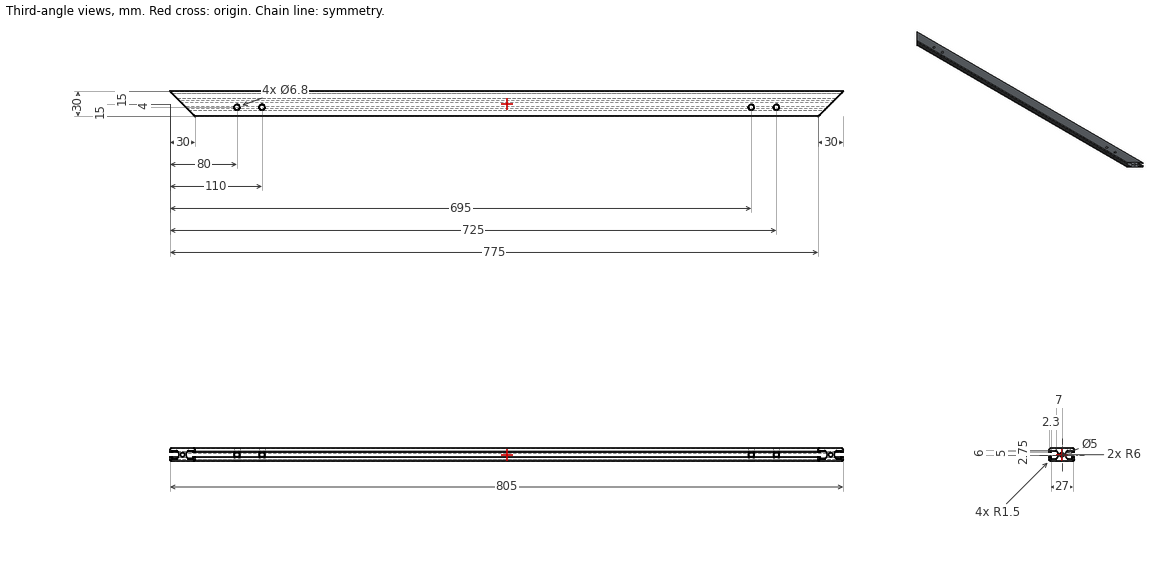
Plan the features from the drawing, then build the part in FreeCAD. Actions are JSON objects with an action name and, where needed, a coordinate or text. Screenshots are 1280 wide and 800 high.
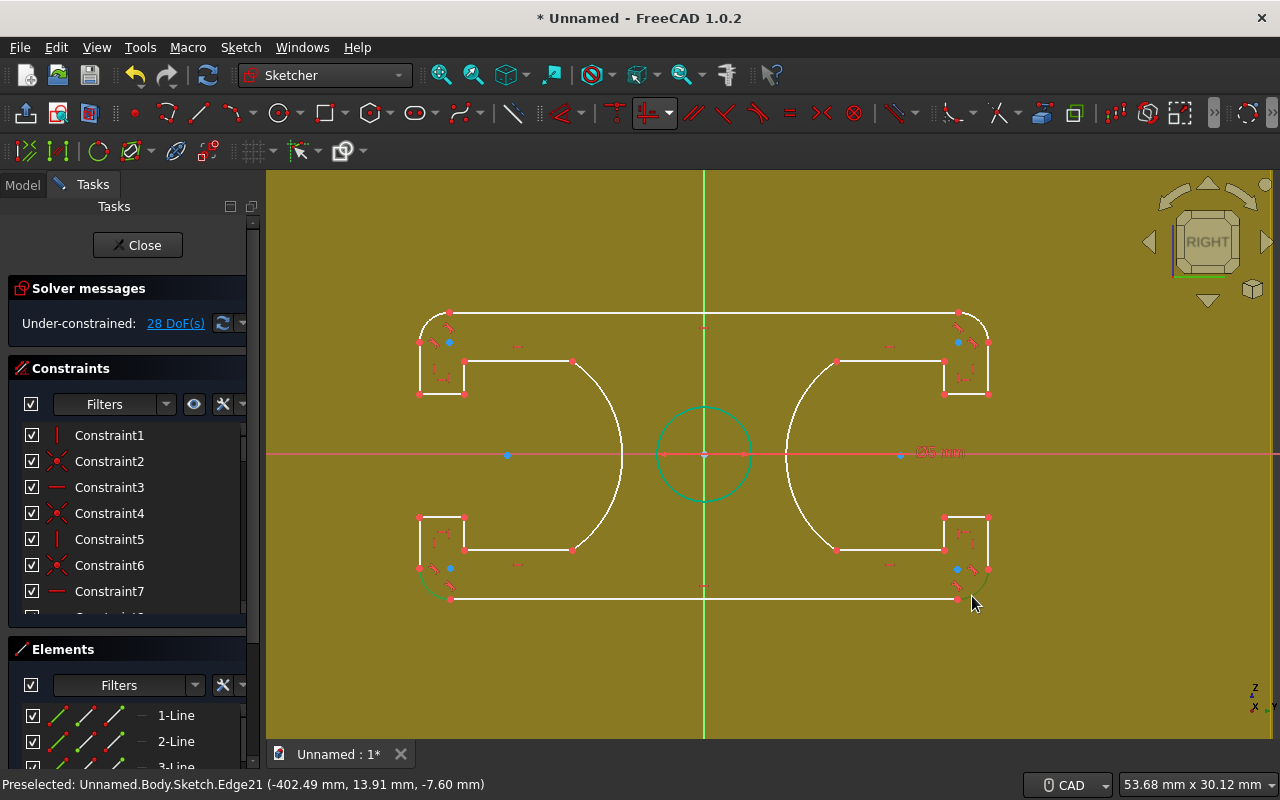
{"action": "left_click", "coordinate": [985, 329]}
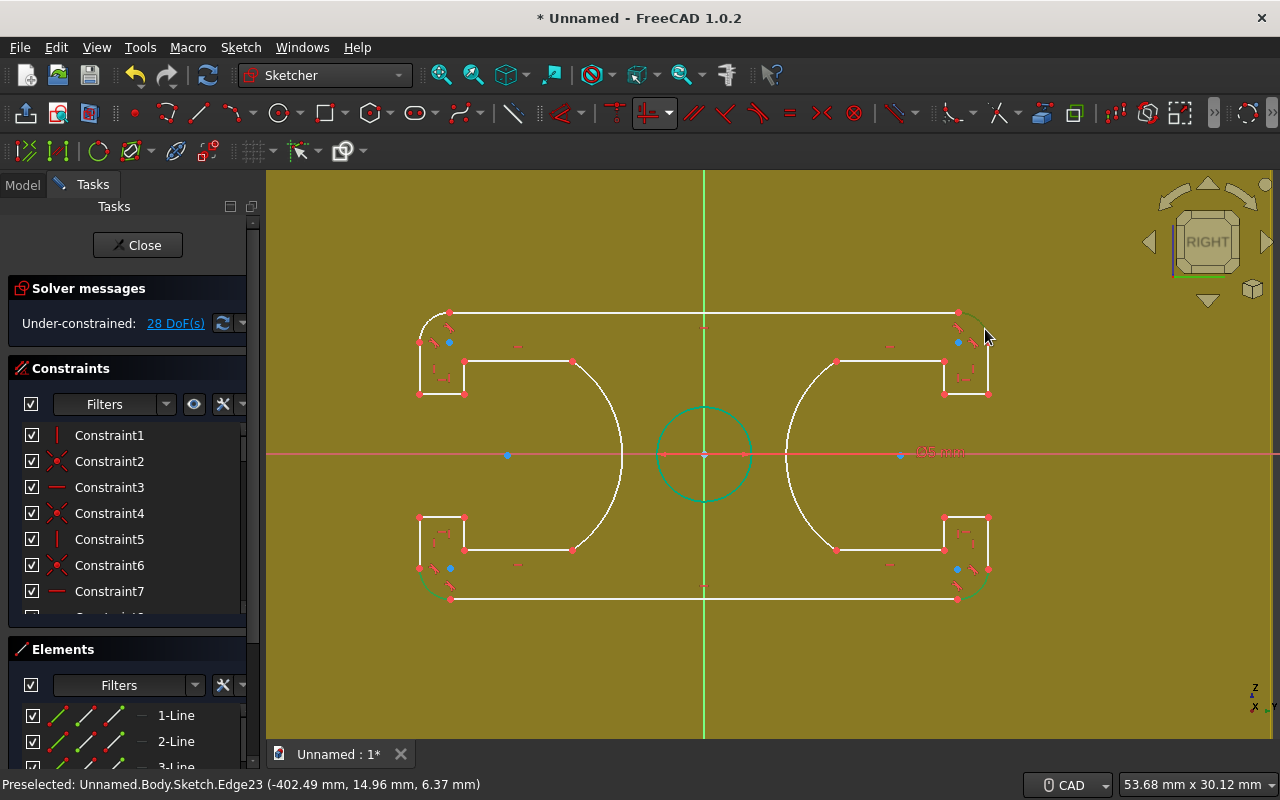
{"action": "left_click", "coordinate": [436, 316]}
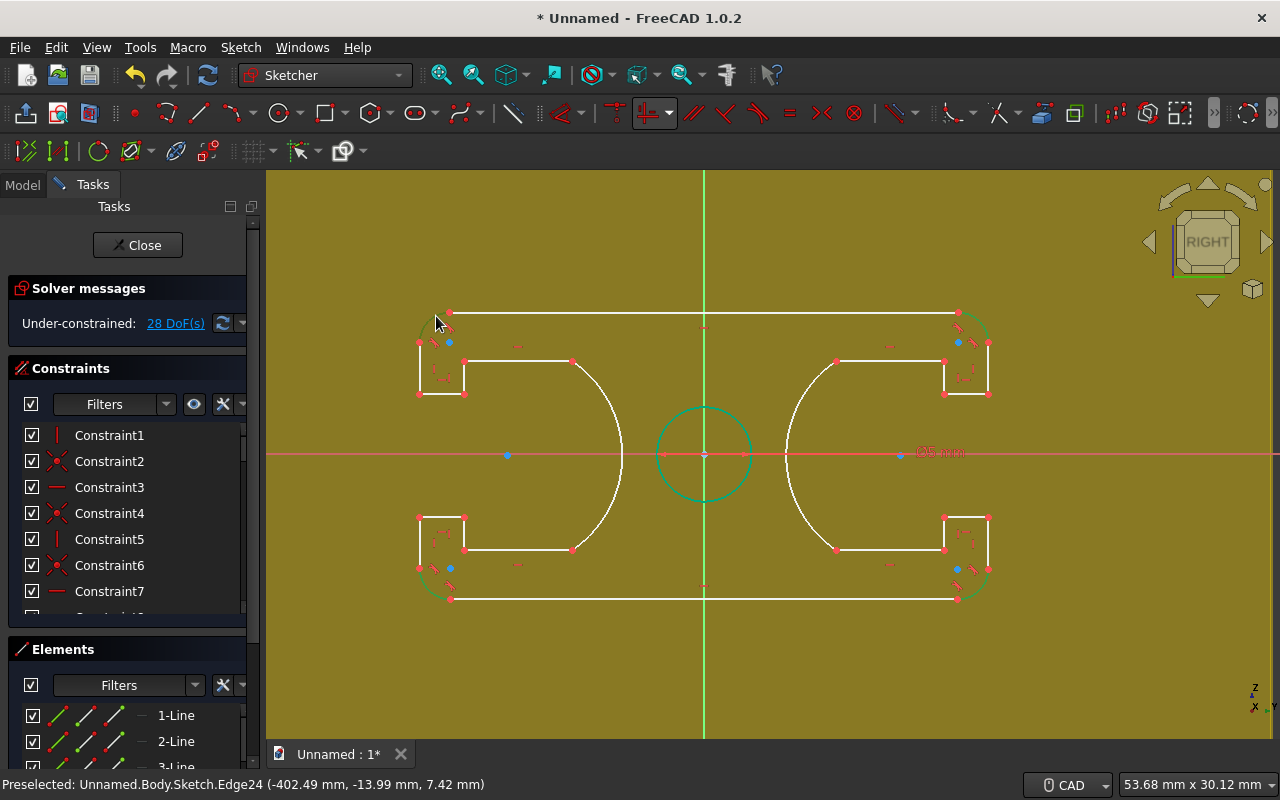
{"action": "left_click", "coordinate": [790, 114]}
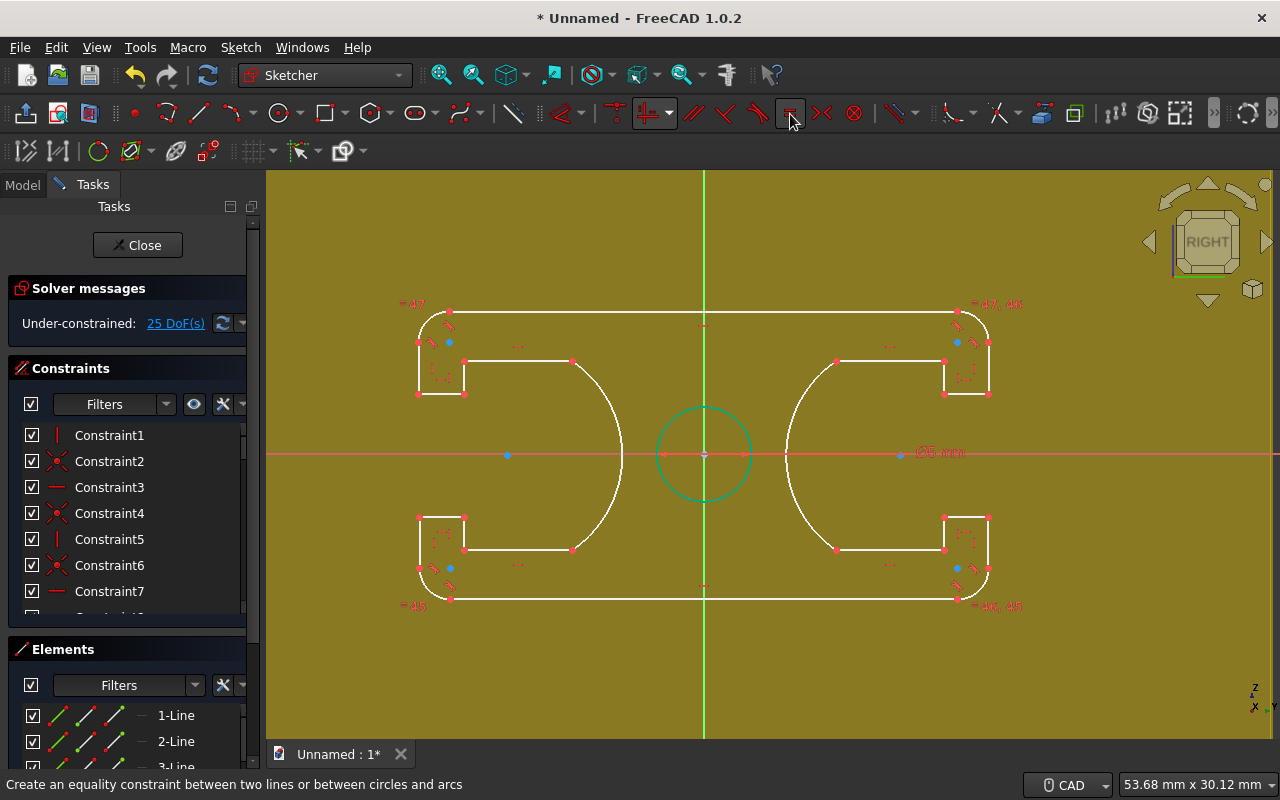
{"action": "left_click", "coordinate": [614, 499]}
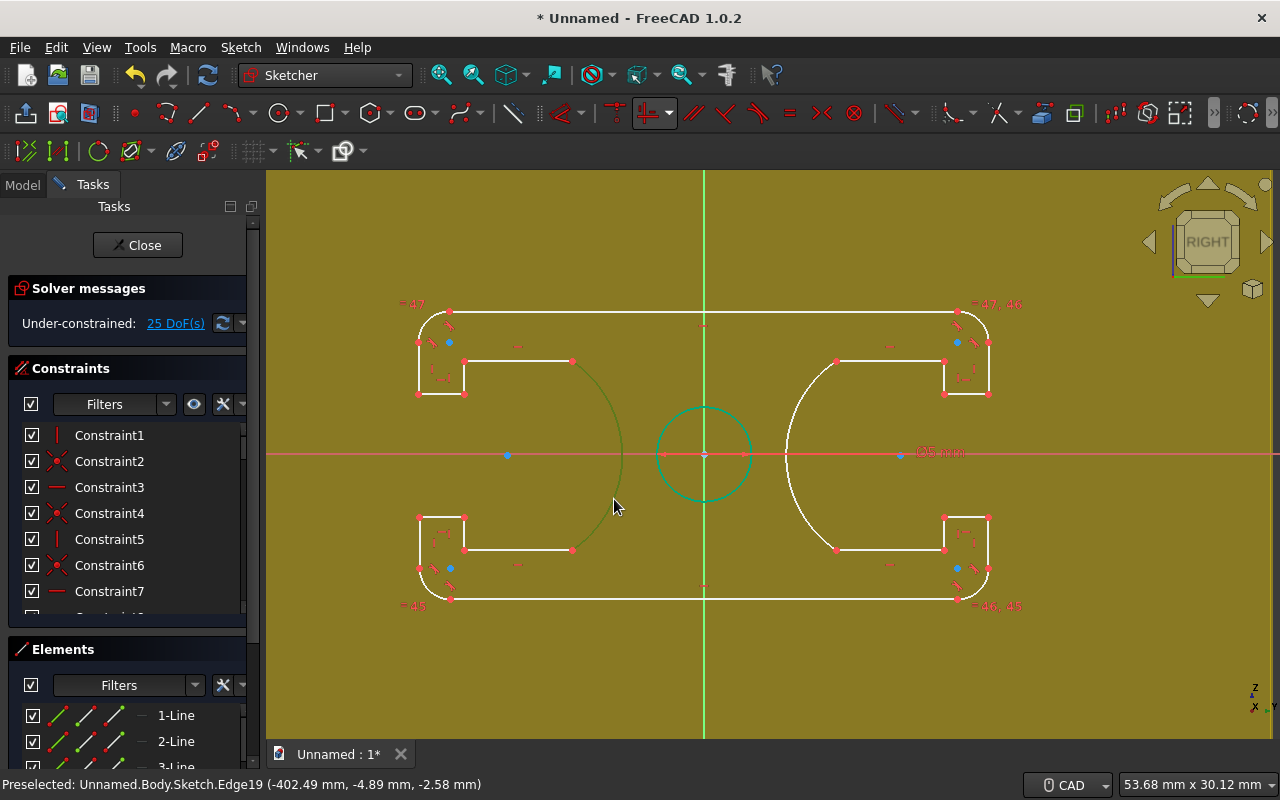
{"action": "left_click", "coordinate": [795, 412]}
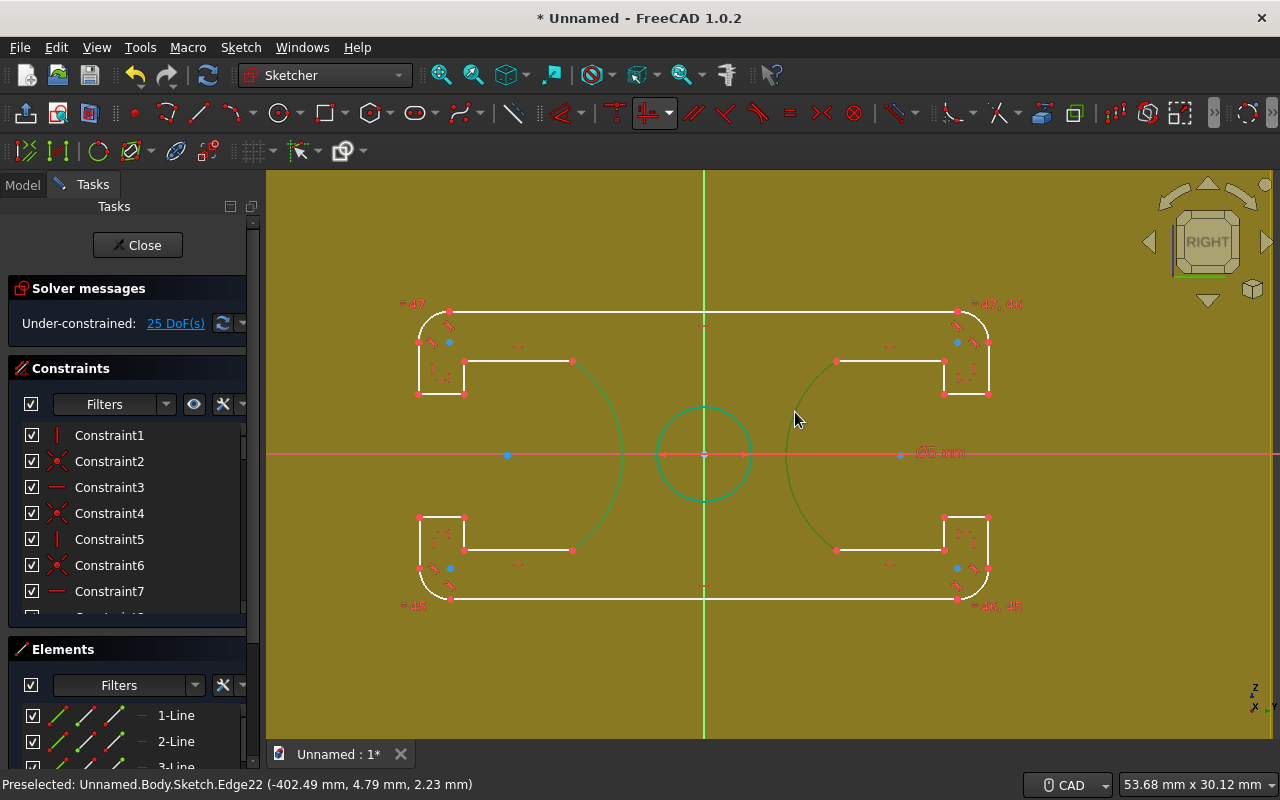
{"action": "left_click", "coordinate": [790, 114]}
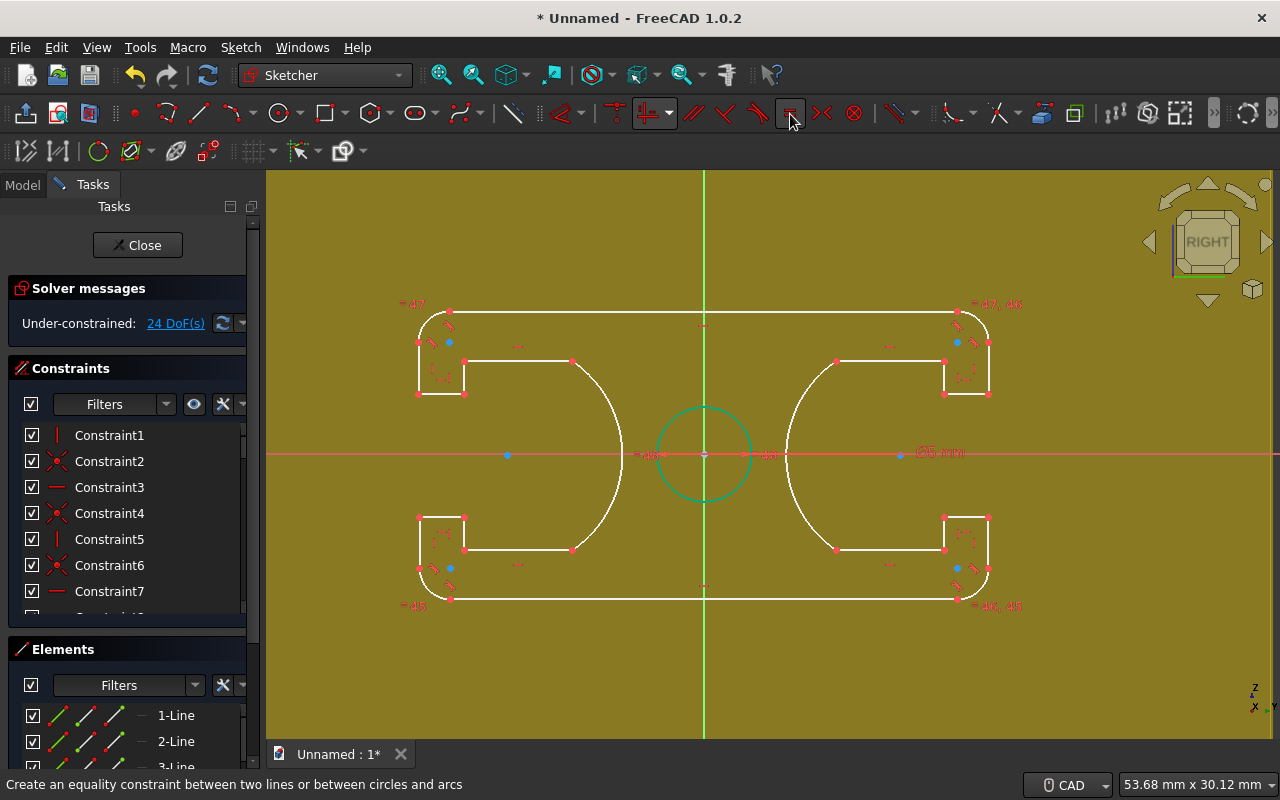
{"action": "left_click", "coordinate": [508, 456]}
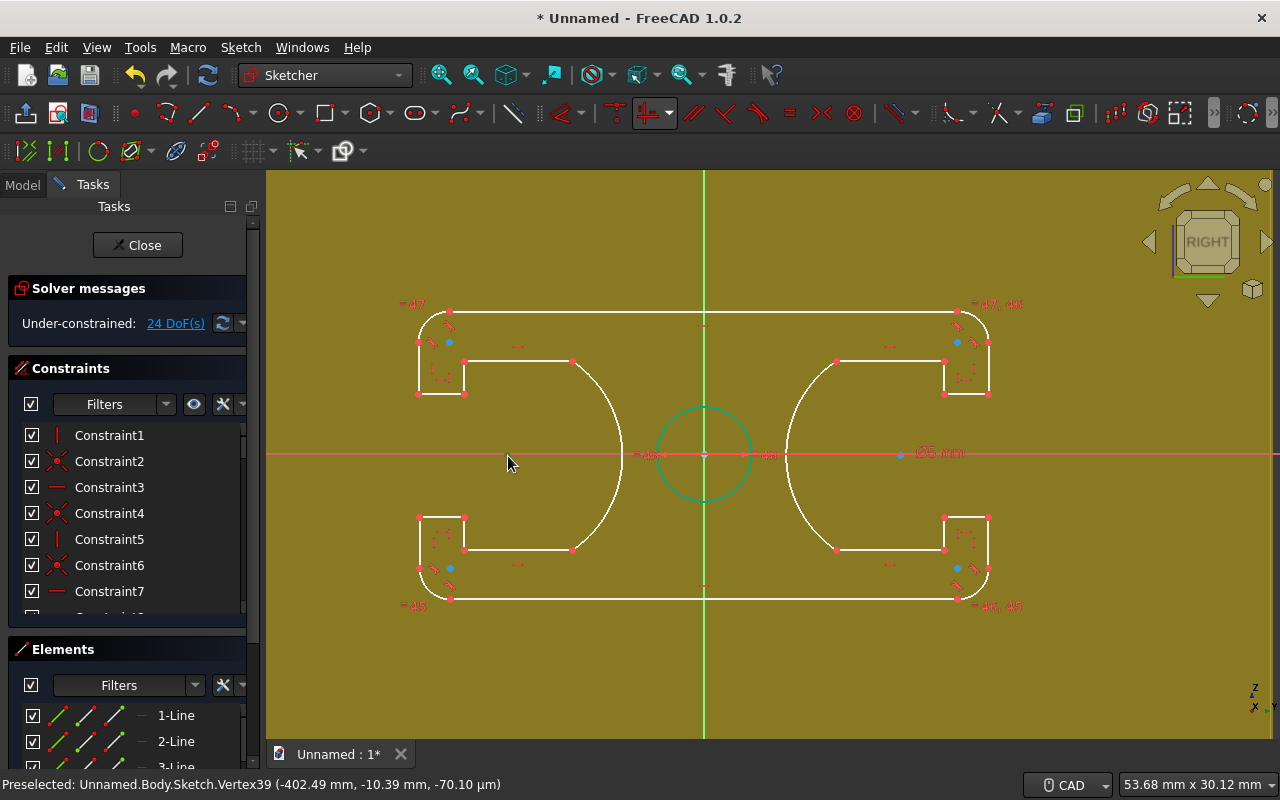
{"action": "left_click", "coordinate": [353, 454]}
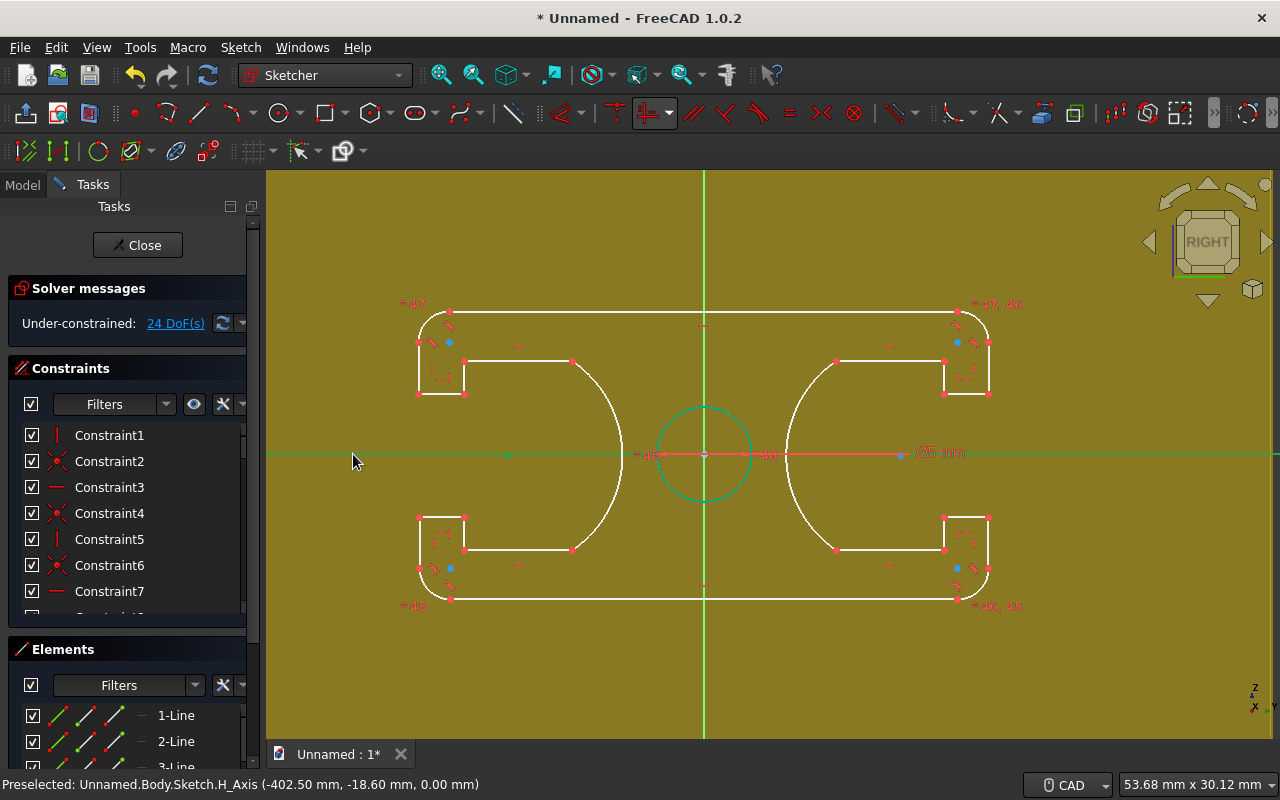
{"action": "left_click", "coordinate": [616, 114]}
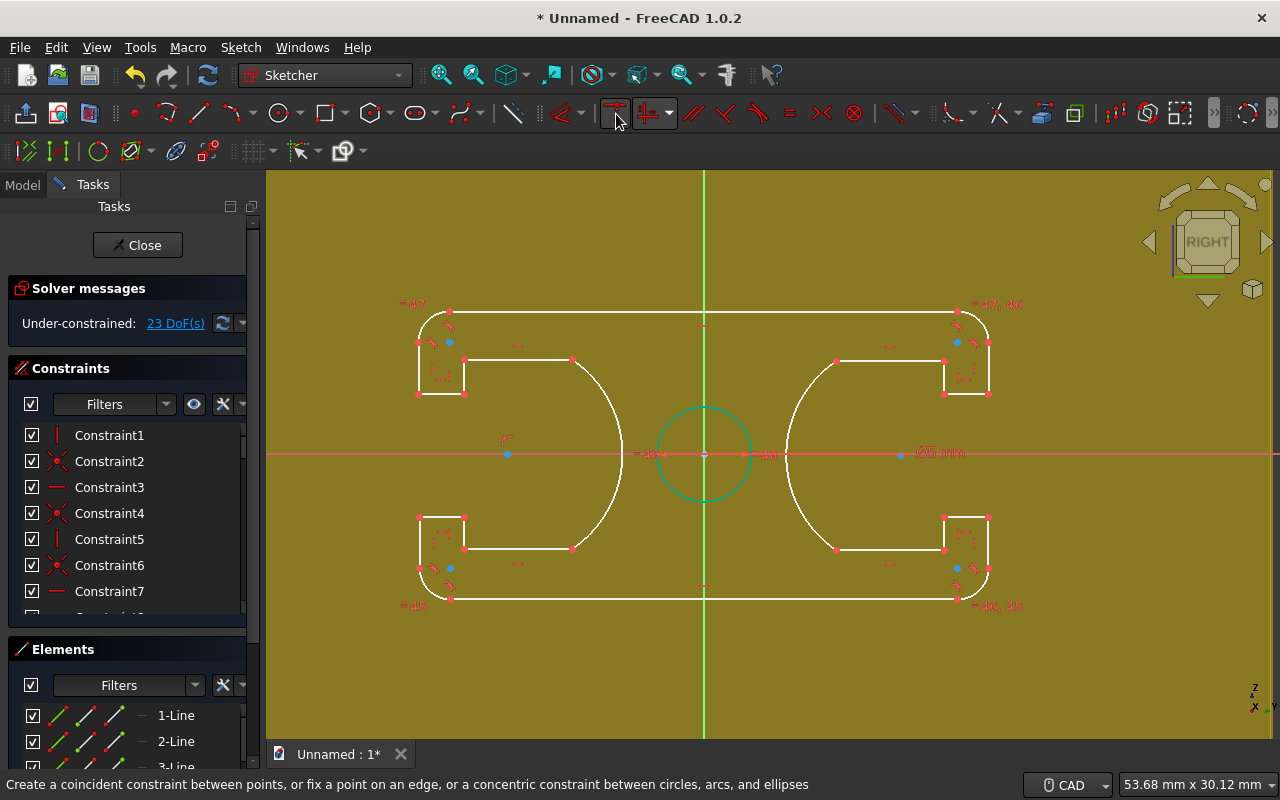
{"action": "left_click", "coordinate": [901, 456]}